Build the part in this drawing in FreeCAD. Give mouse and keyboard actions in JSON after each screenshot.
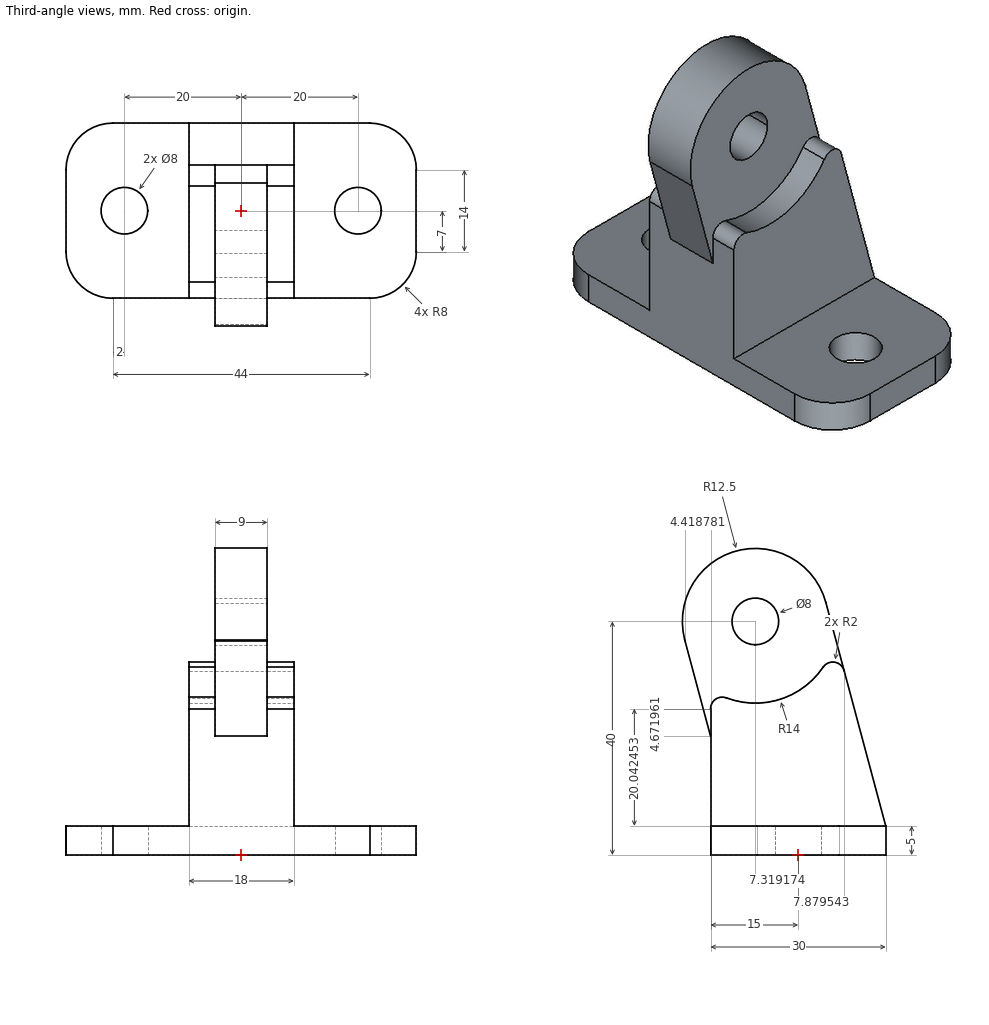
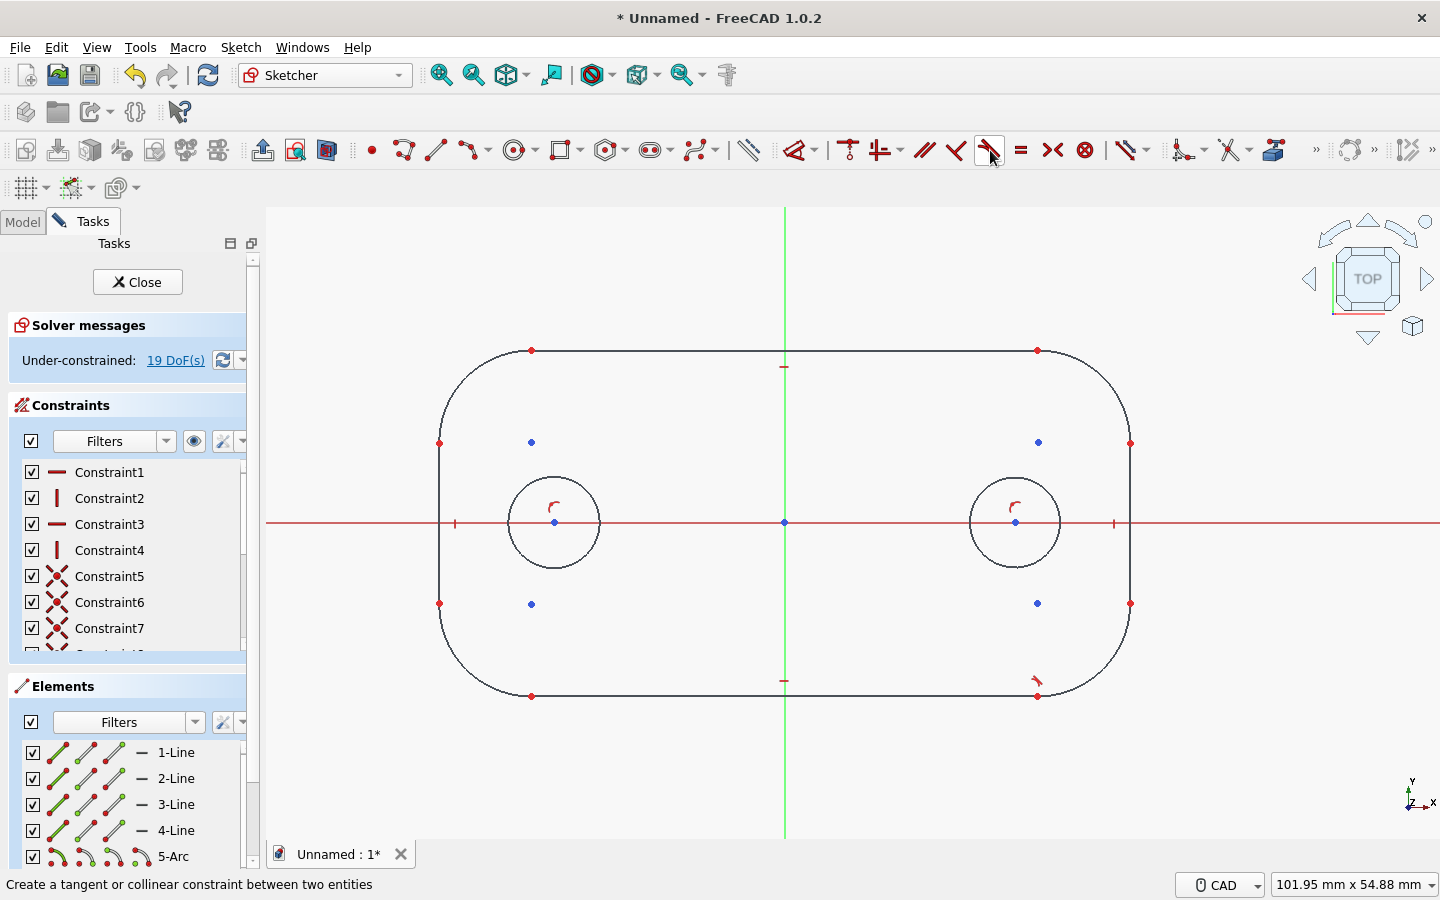
{"action": "left_click", "coordinate": [683, 696]}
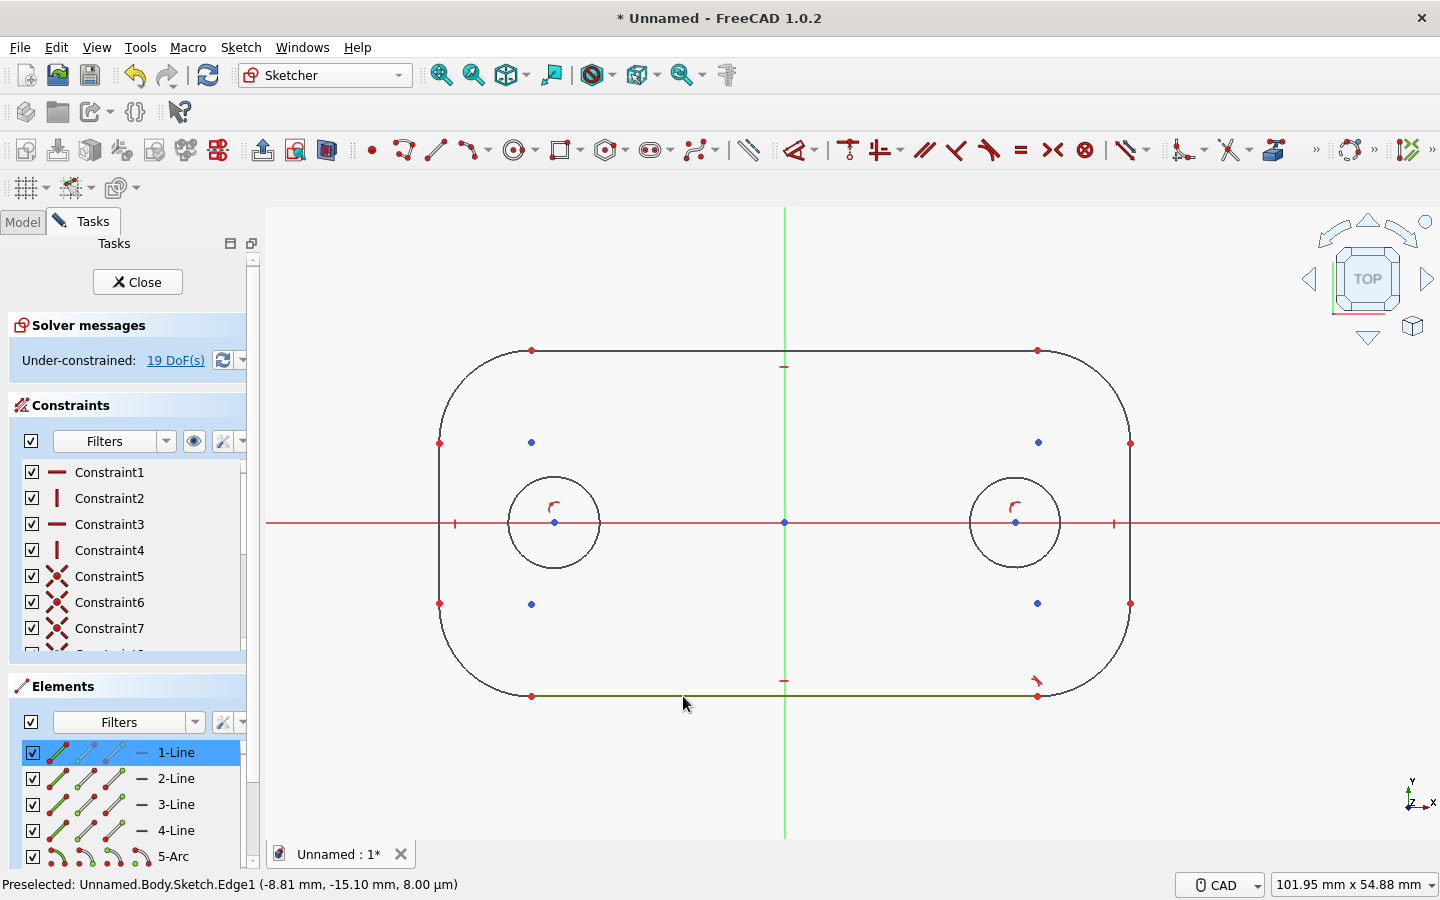
{"action": "left_click", "coordinate": [449, 646]}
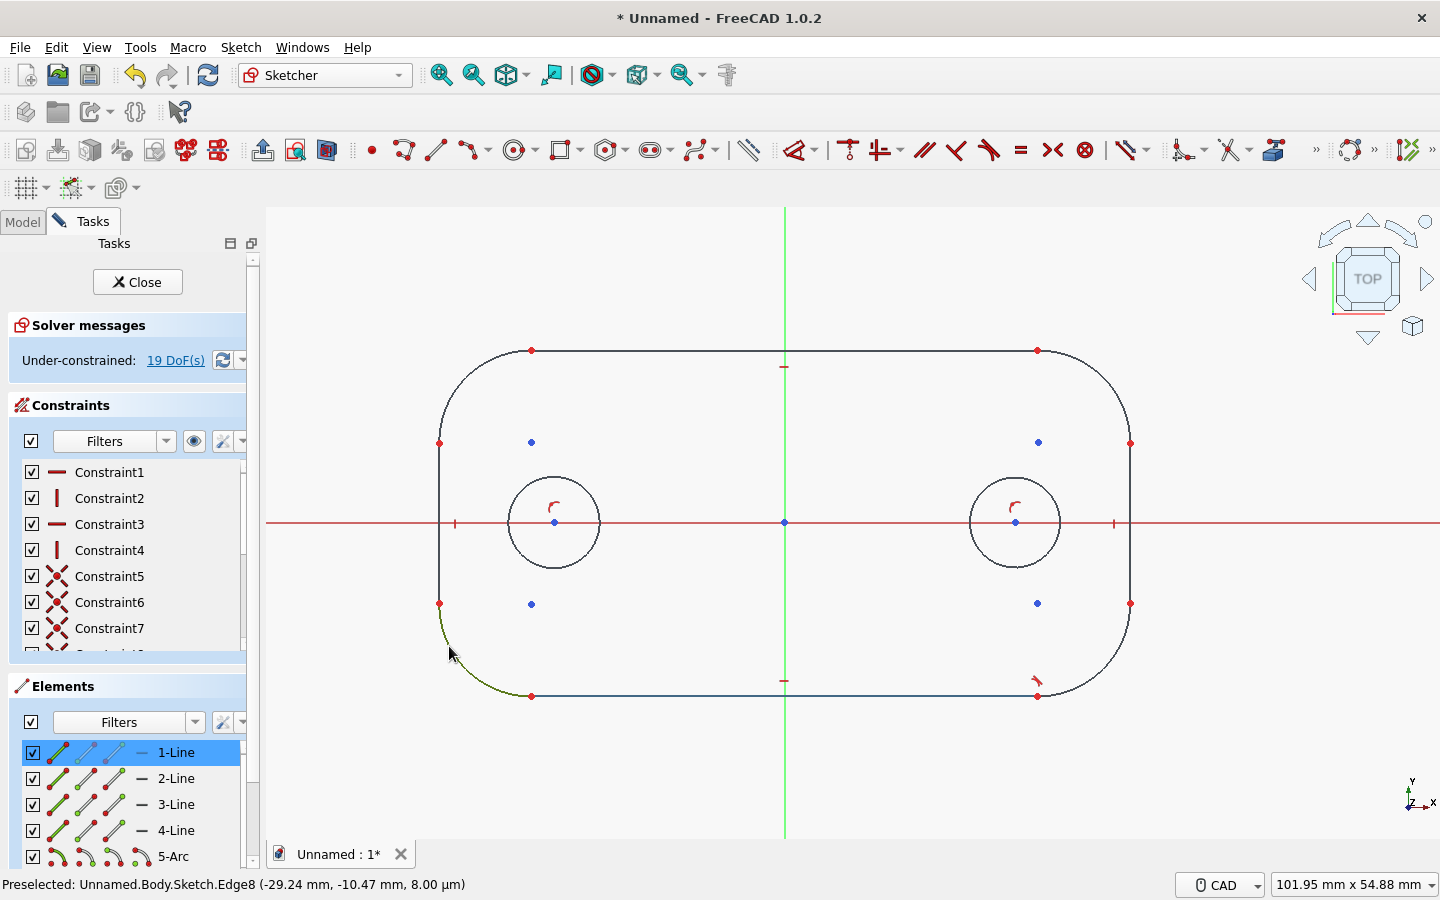
{"action": "key", "text": "t"}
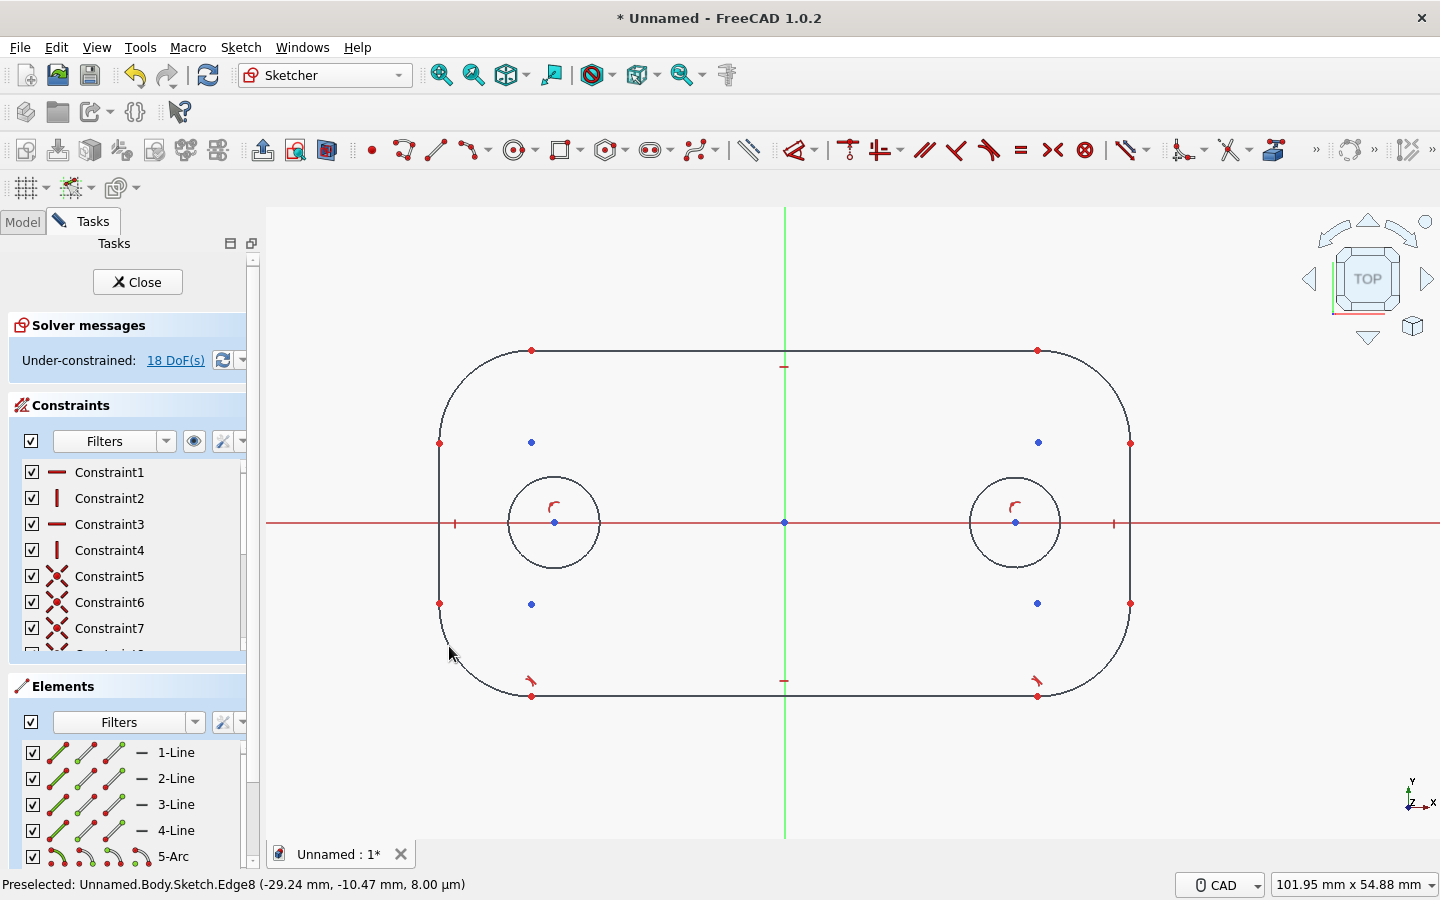
{"action": "left_click", "coordinate": [1130, 556]}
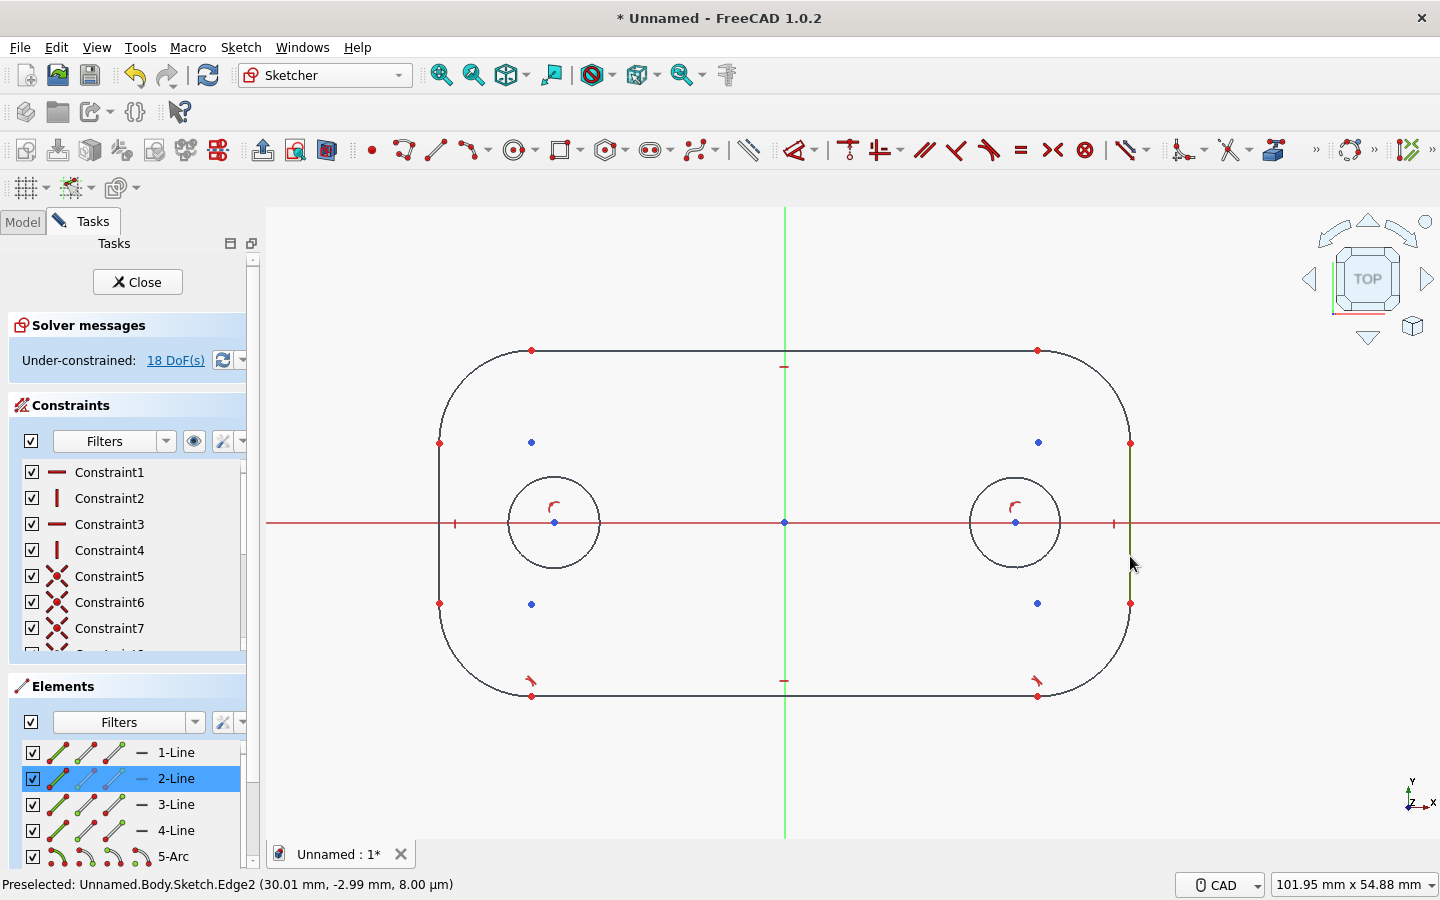
{"action": "left_click", "coordinate": [1080, 686]}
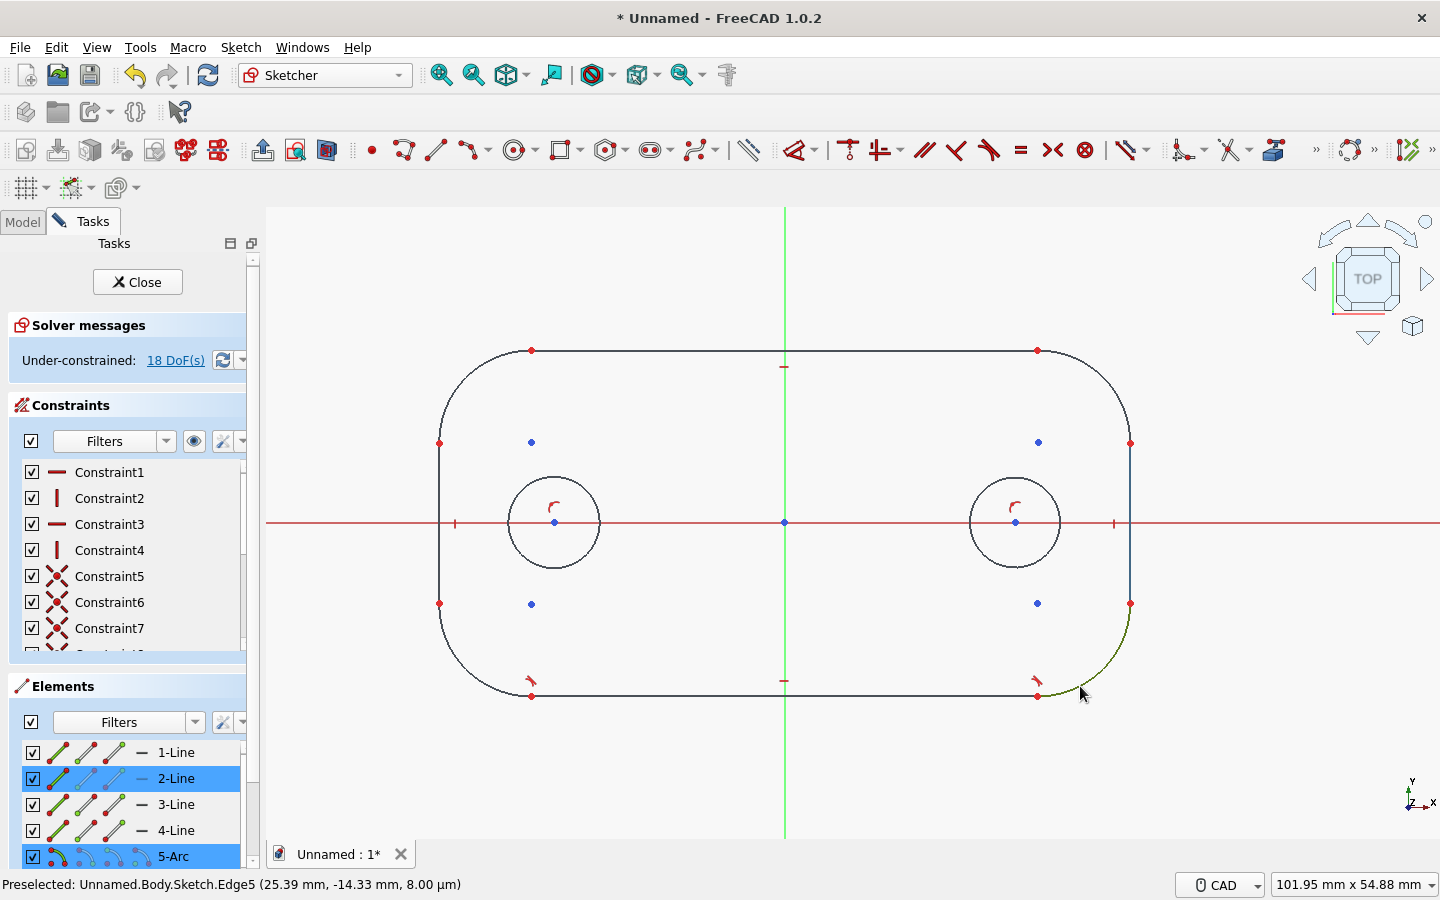
{"action": "left_click", "coordinate": [990, 150]}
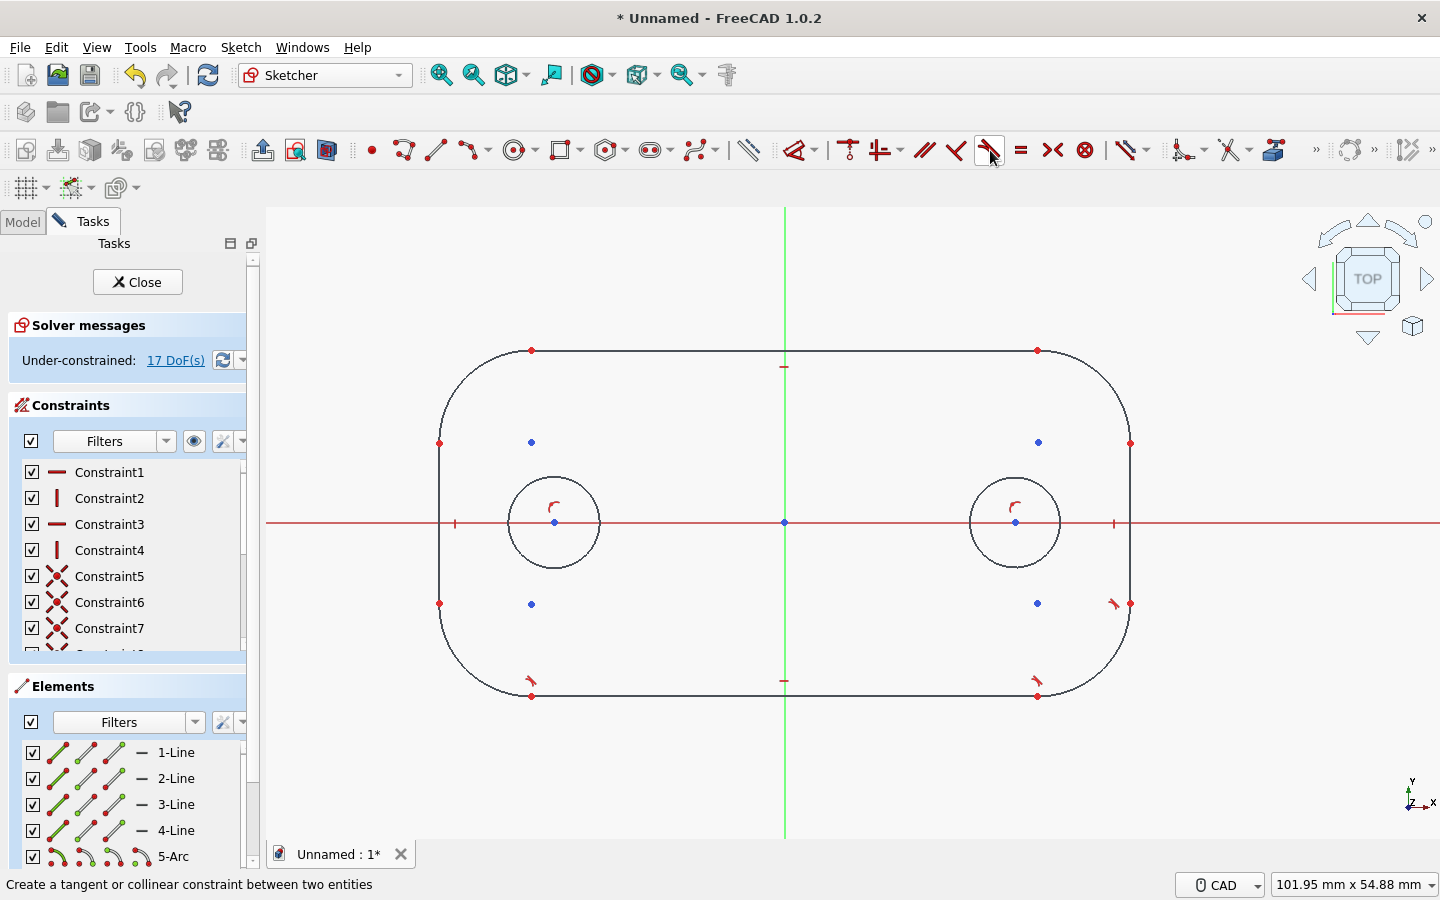
{"action": "left_click", "coordinate": [1130, 556]}